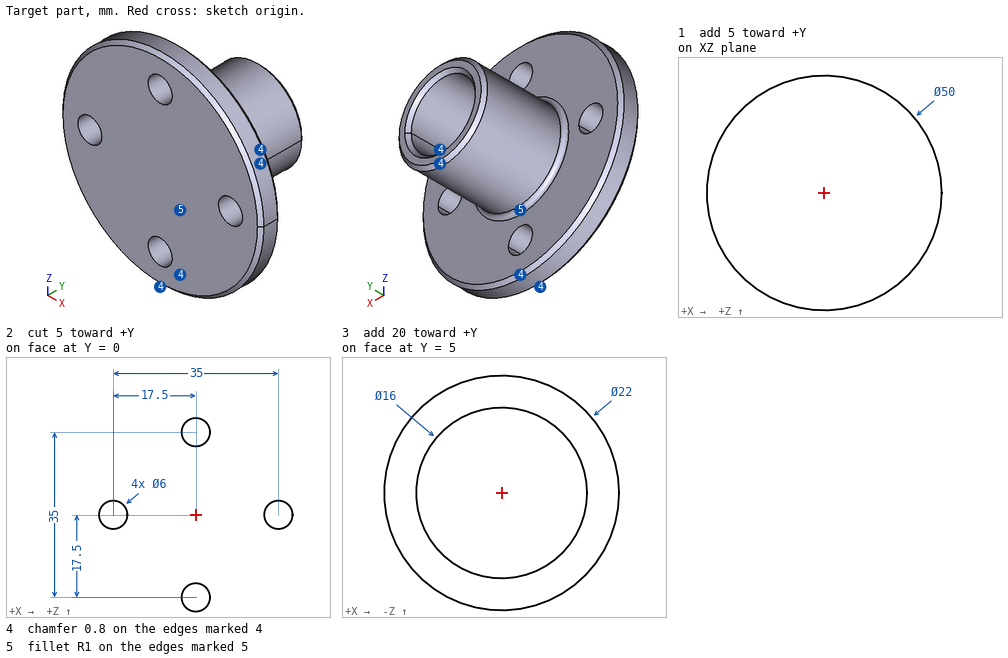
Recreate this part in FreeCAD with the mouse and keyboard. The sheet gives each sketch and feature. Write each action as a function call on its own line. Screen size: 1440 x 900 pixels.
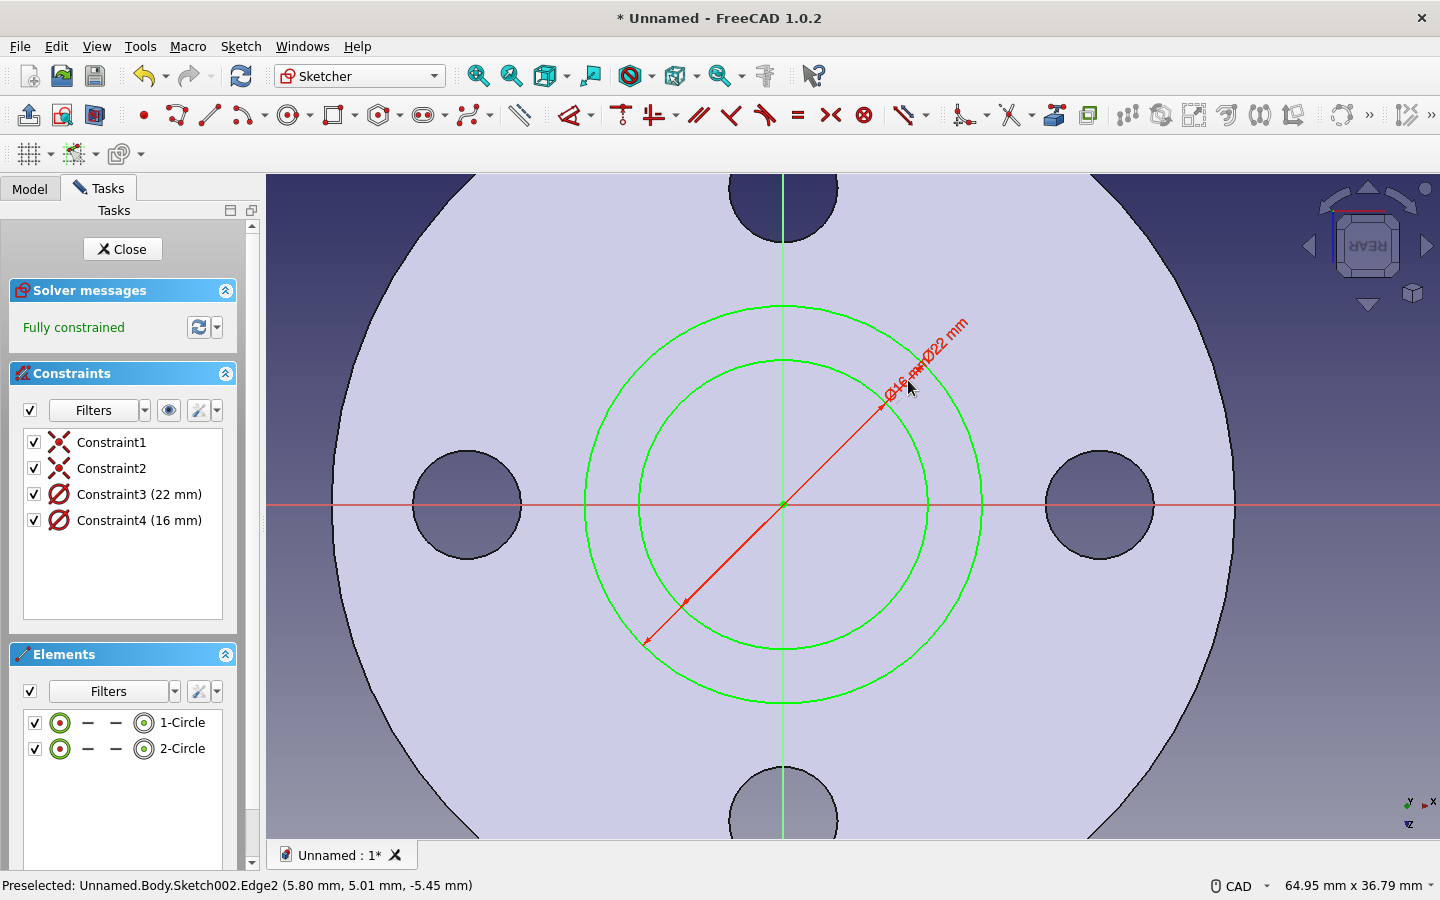
click(123, 249)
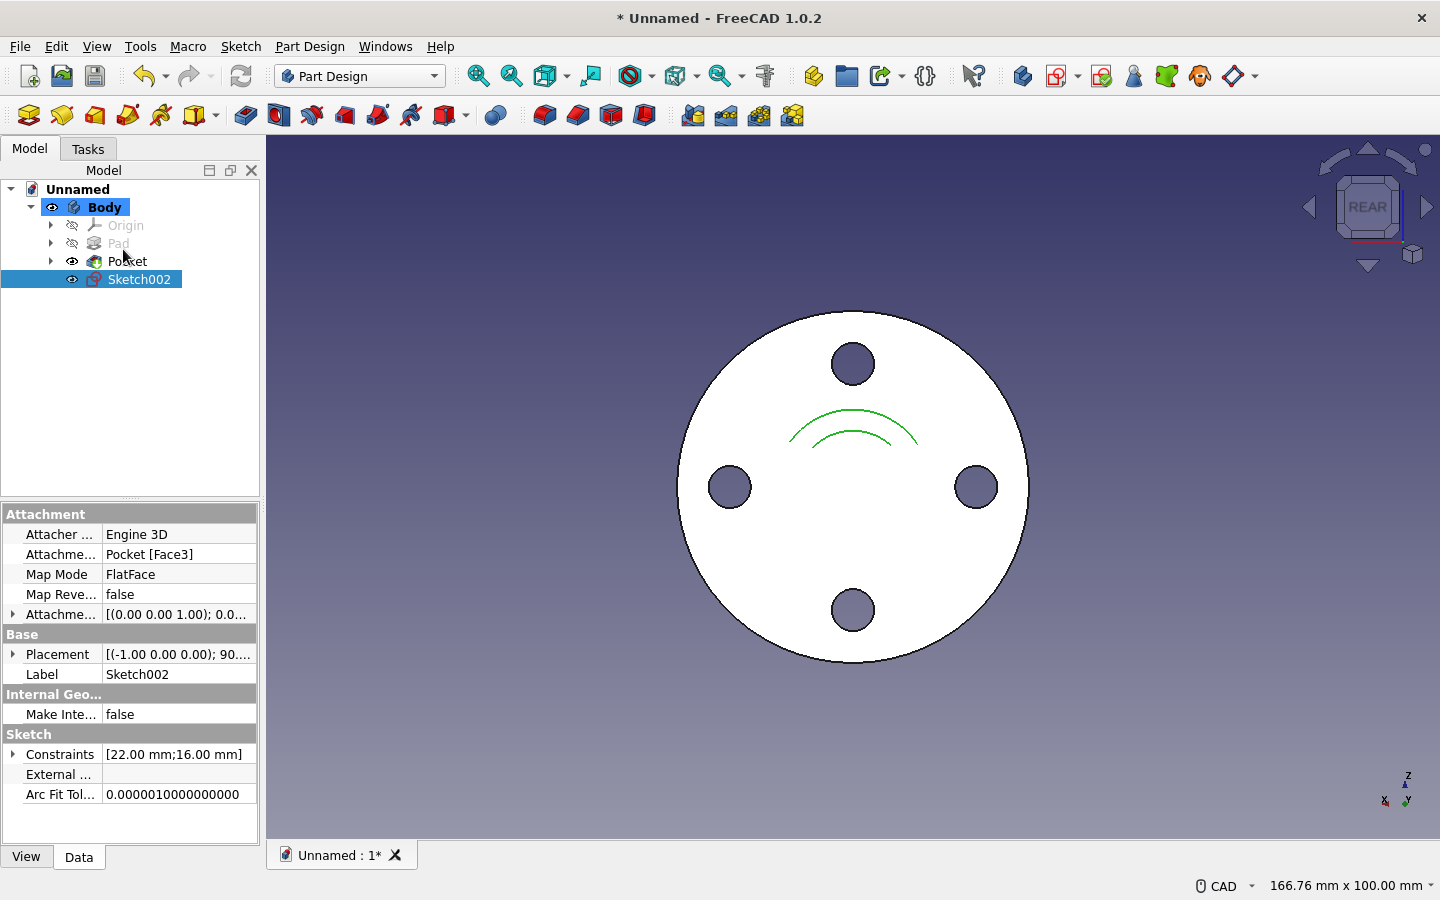
click(29, 116)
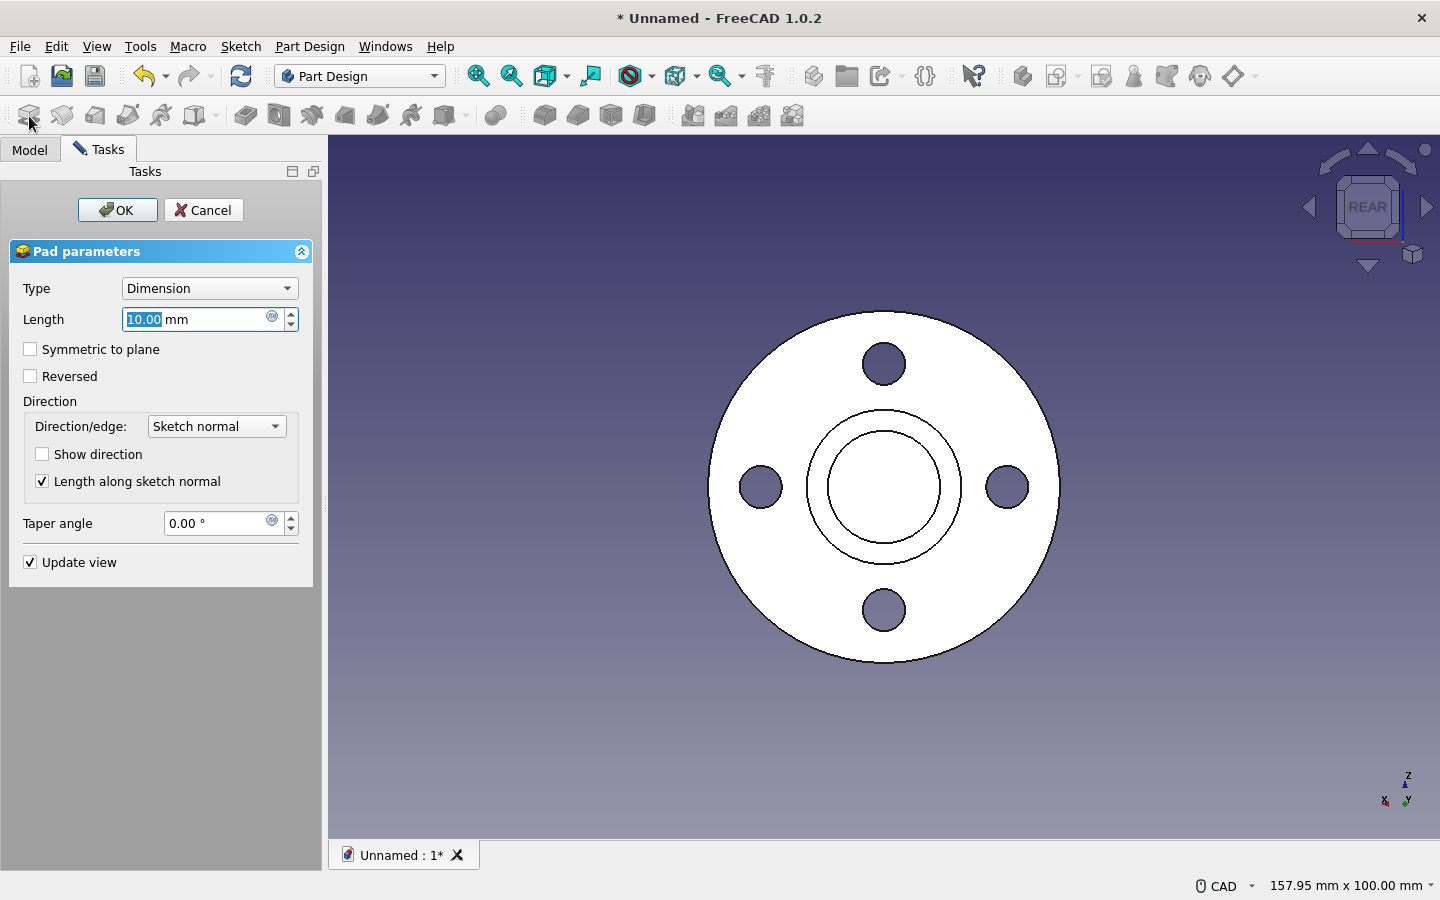
text(20)
key(Tab)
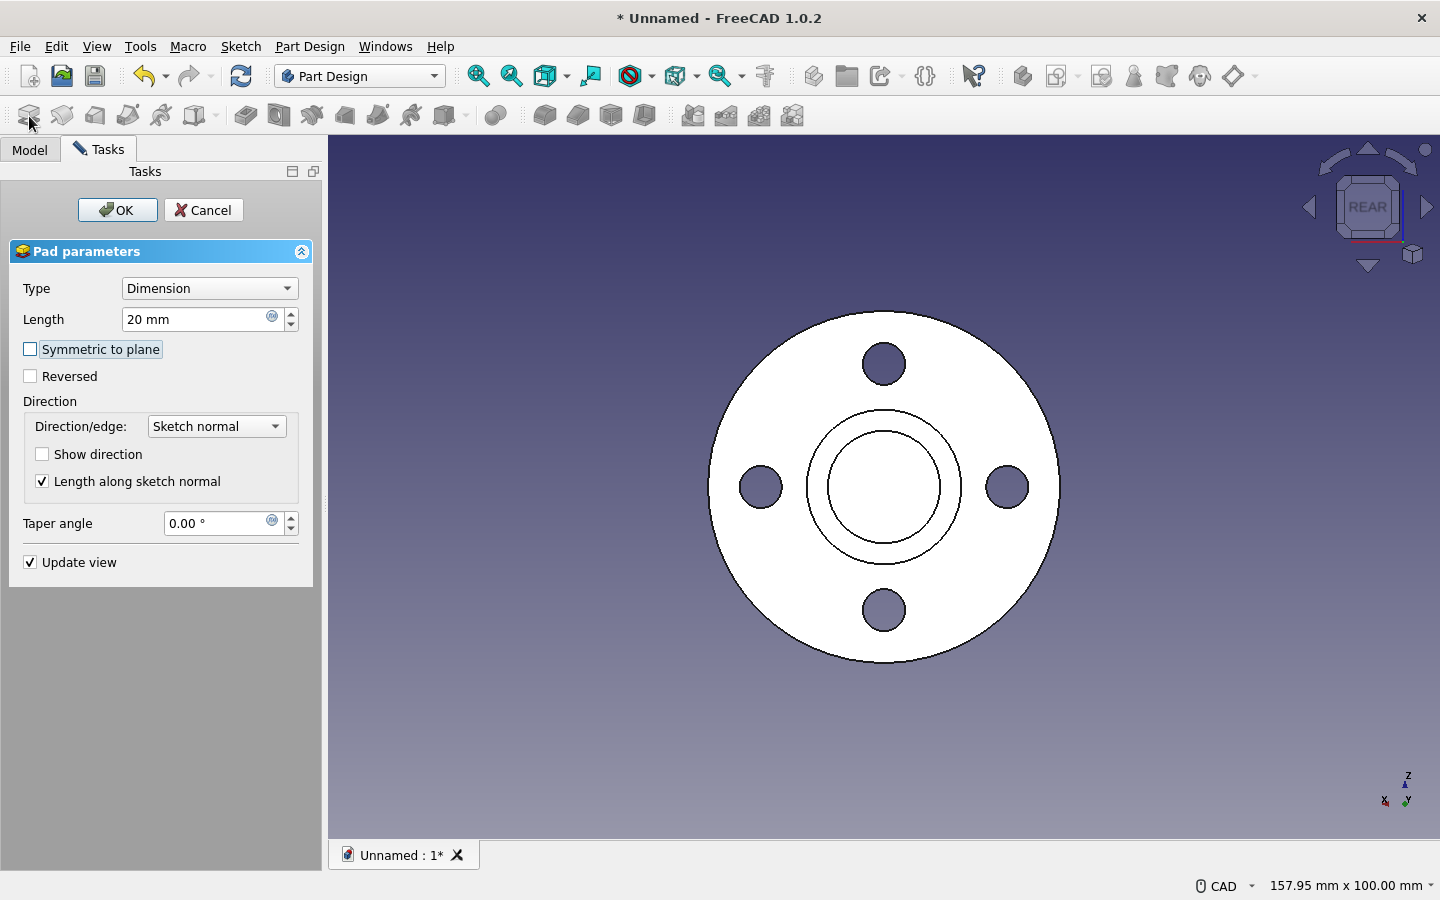
click(118, 210)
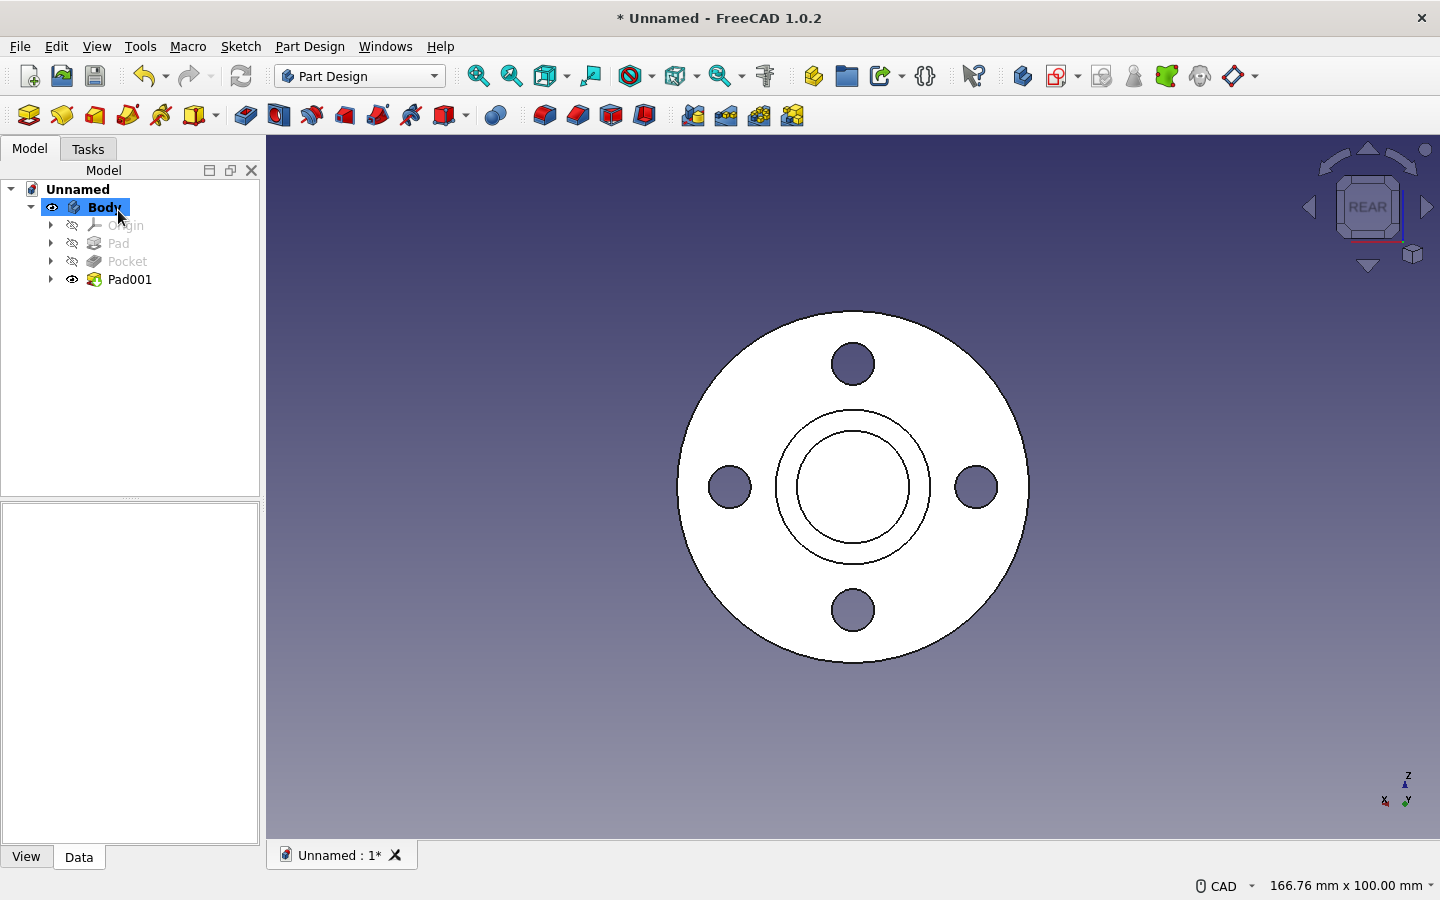
click(930, 486)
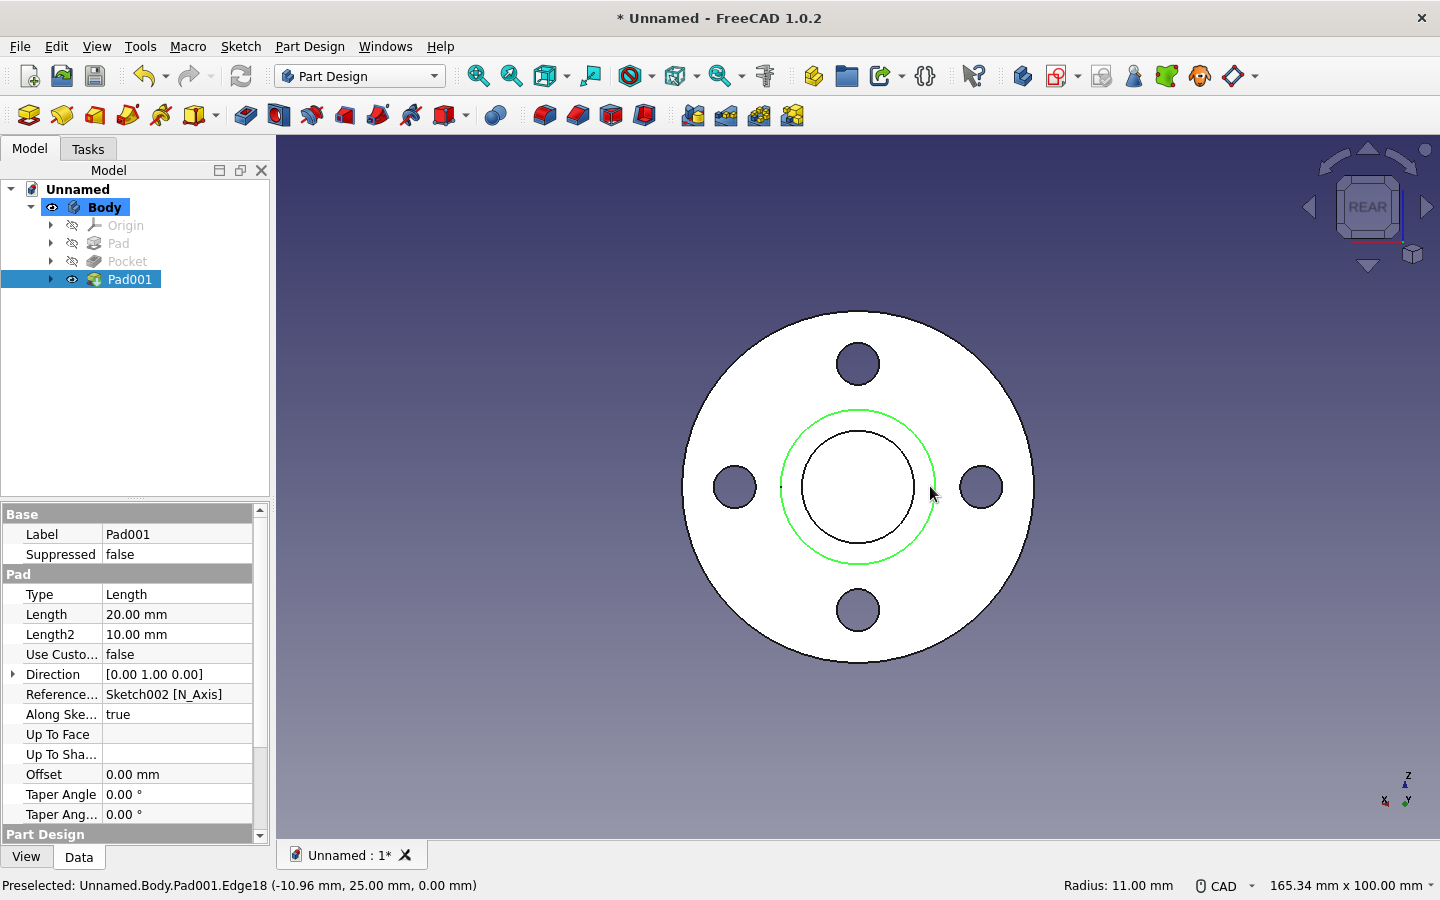
click(904, 453, ctrl)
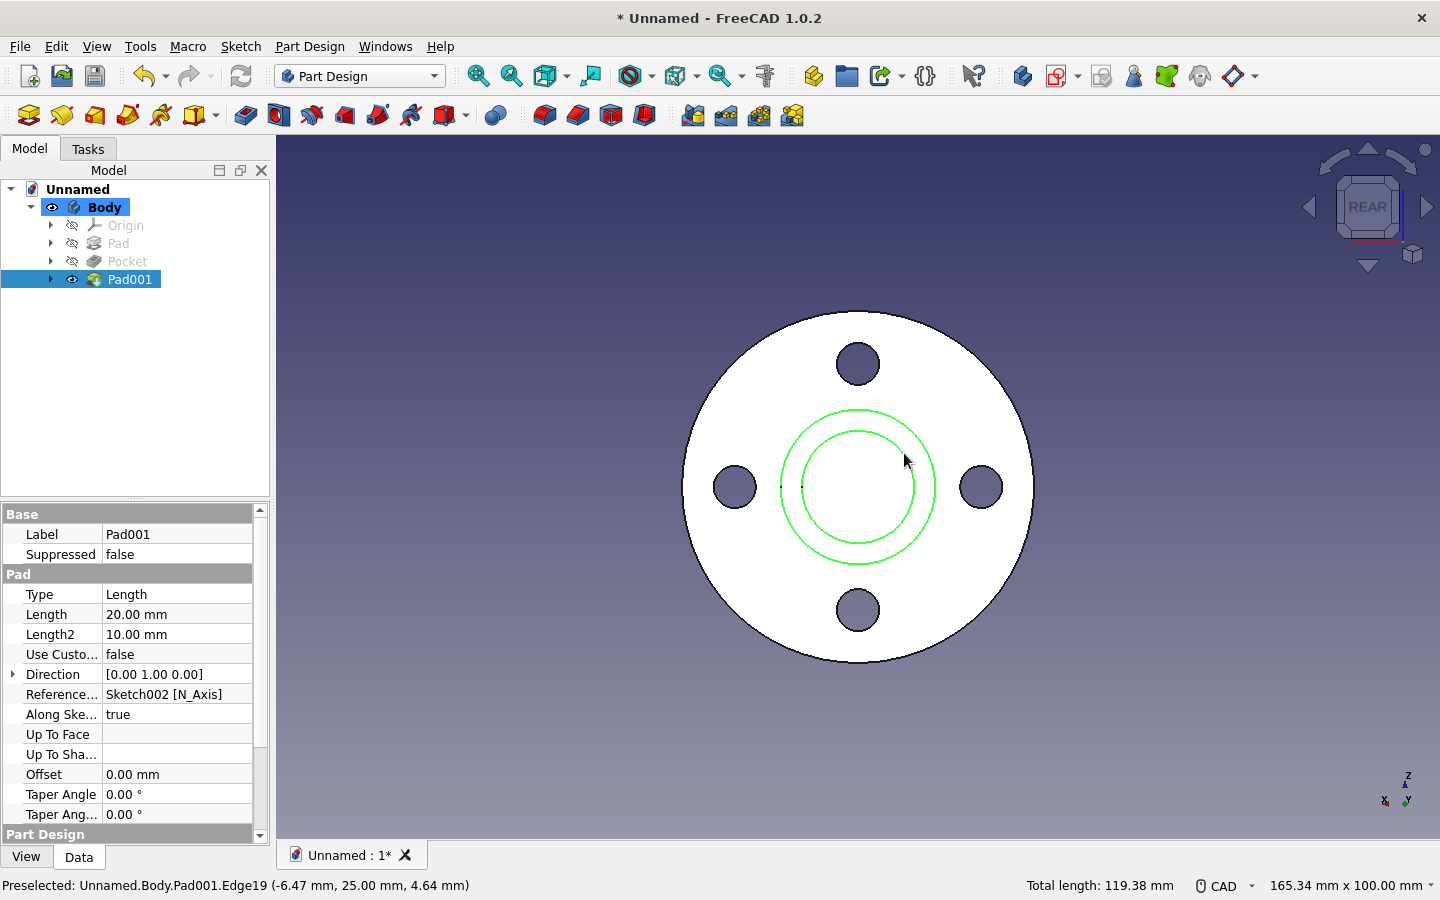
click(1034, 486, ctrl)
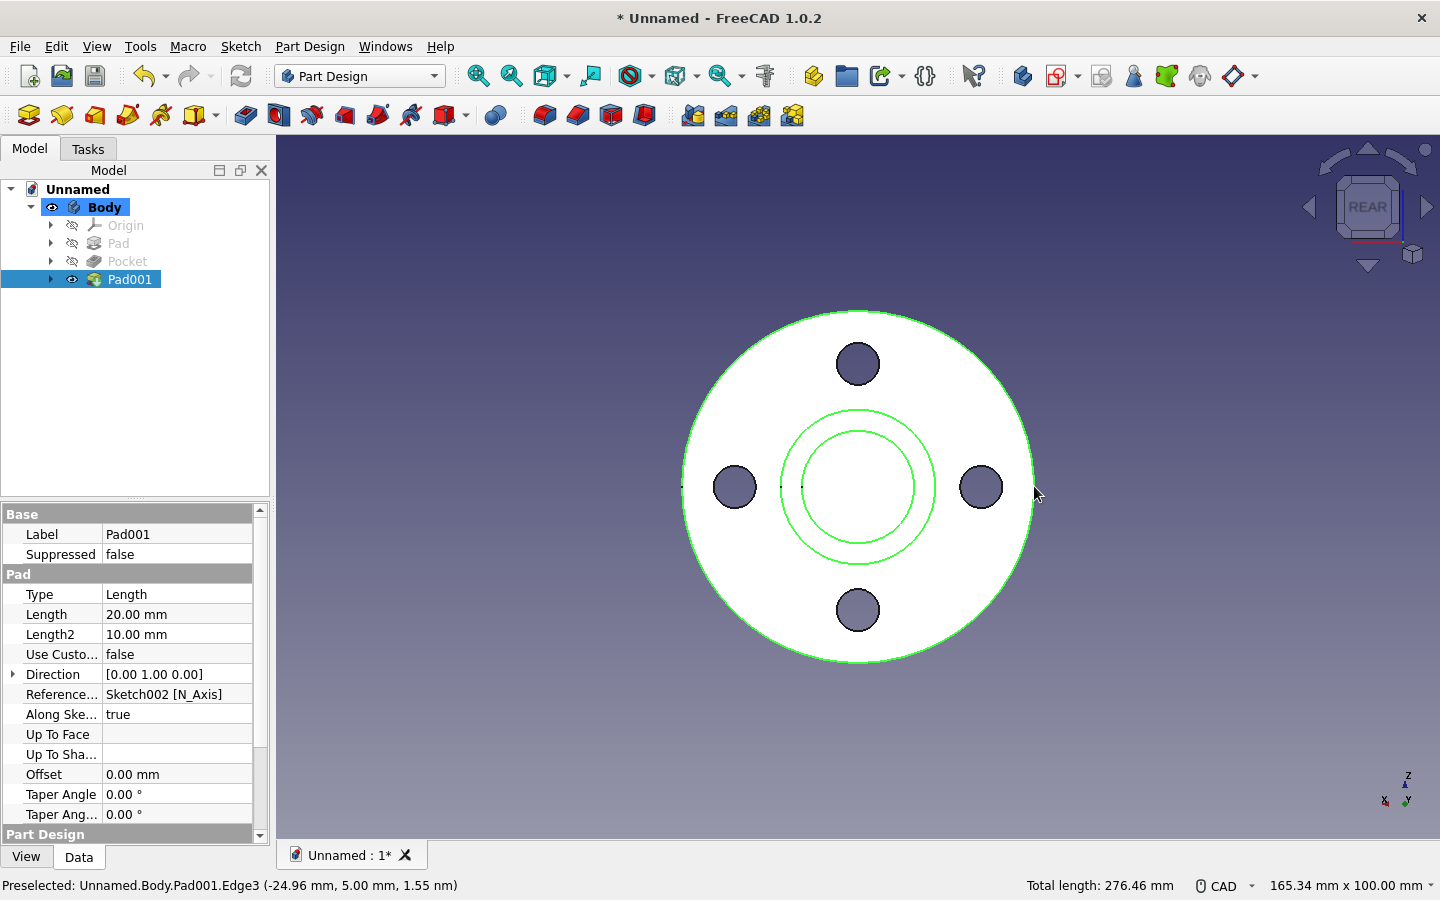
key(0)